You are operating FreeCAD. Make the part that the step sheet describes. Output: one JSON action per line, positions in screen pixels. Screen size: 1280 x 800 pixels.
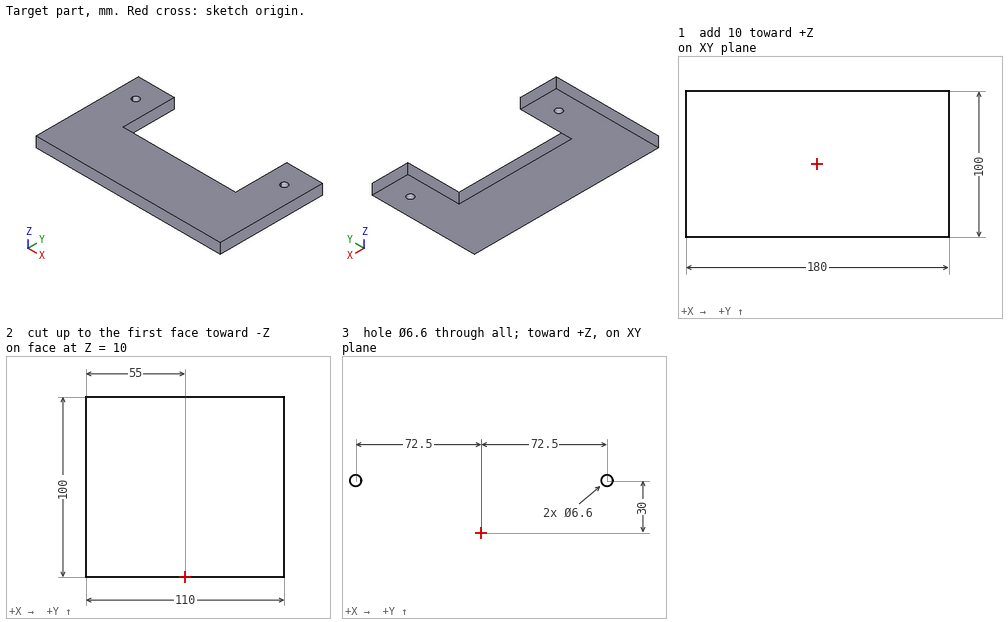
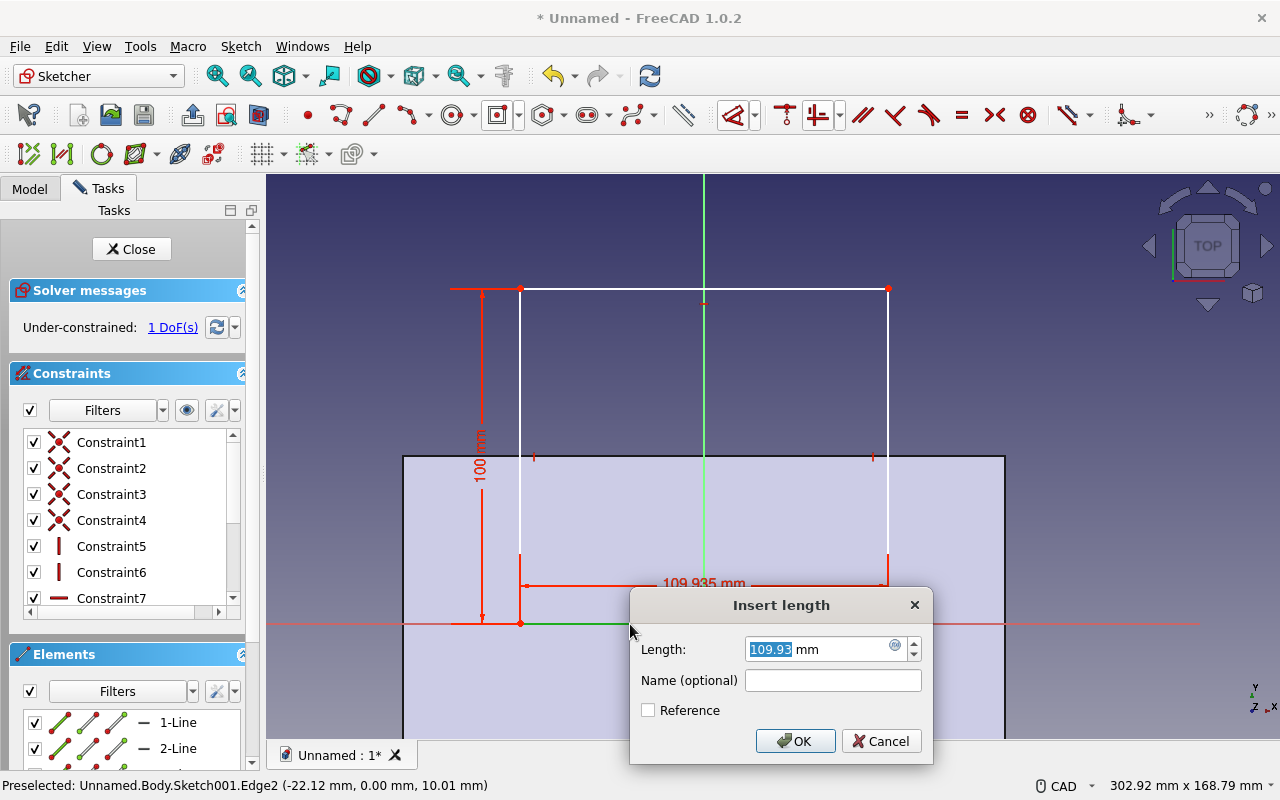
{"action": "type", "text": "110"}
{"action": "key", "text": "Return"}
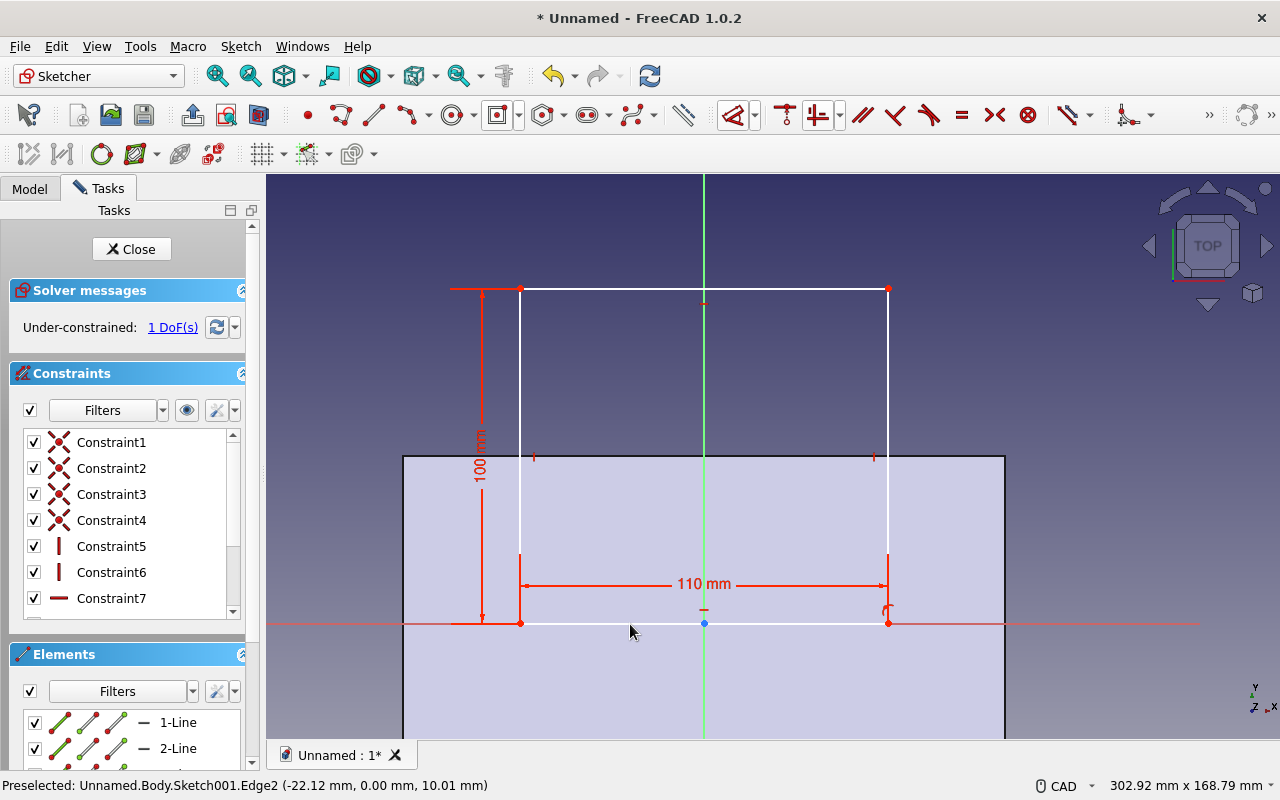
{"action": "left_click", "coordinate": [520, 289]}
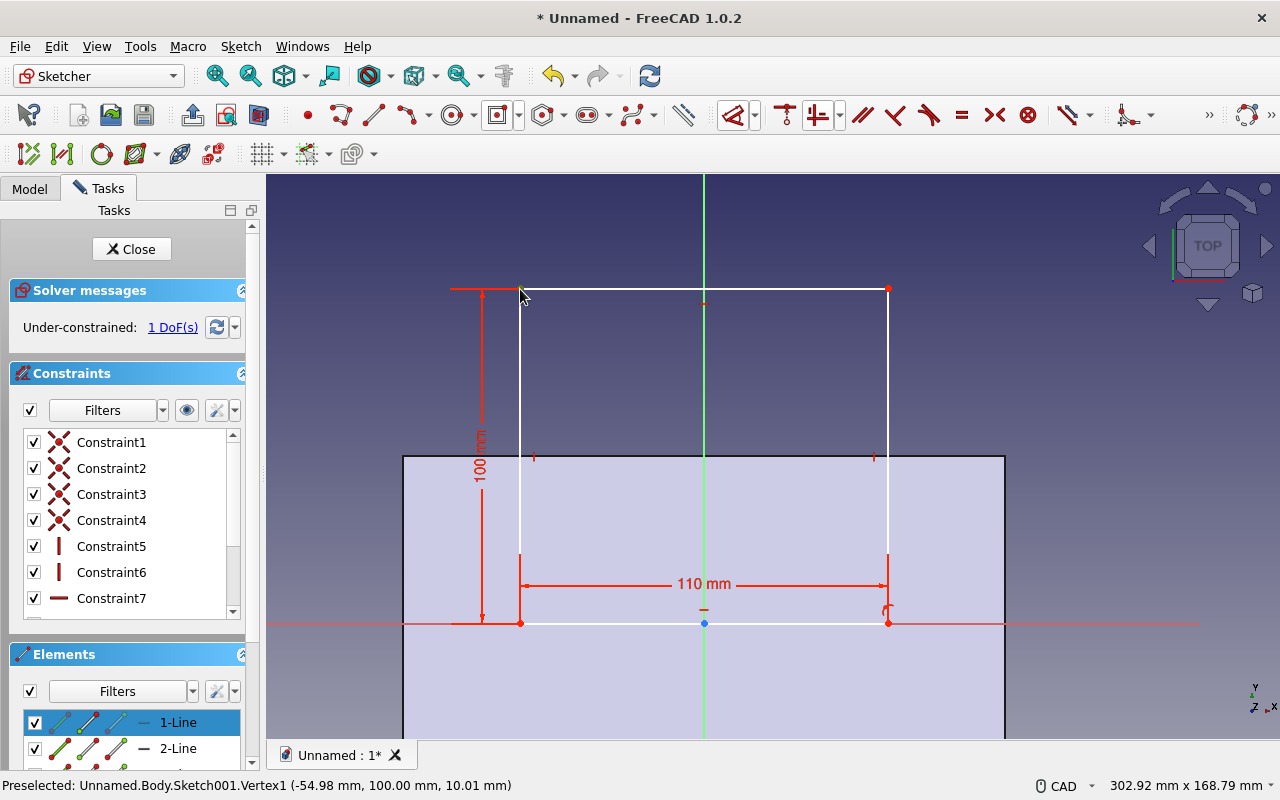
{"action": "key", "text": "l"}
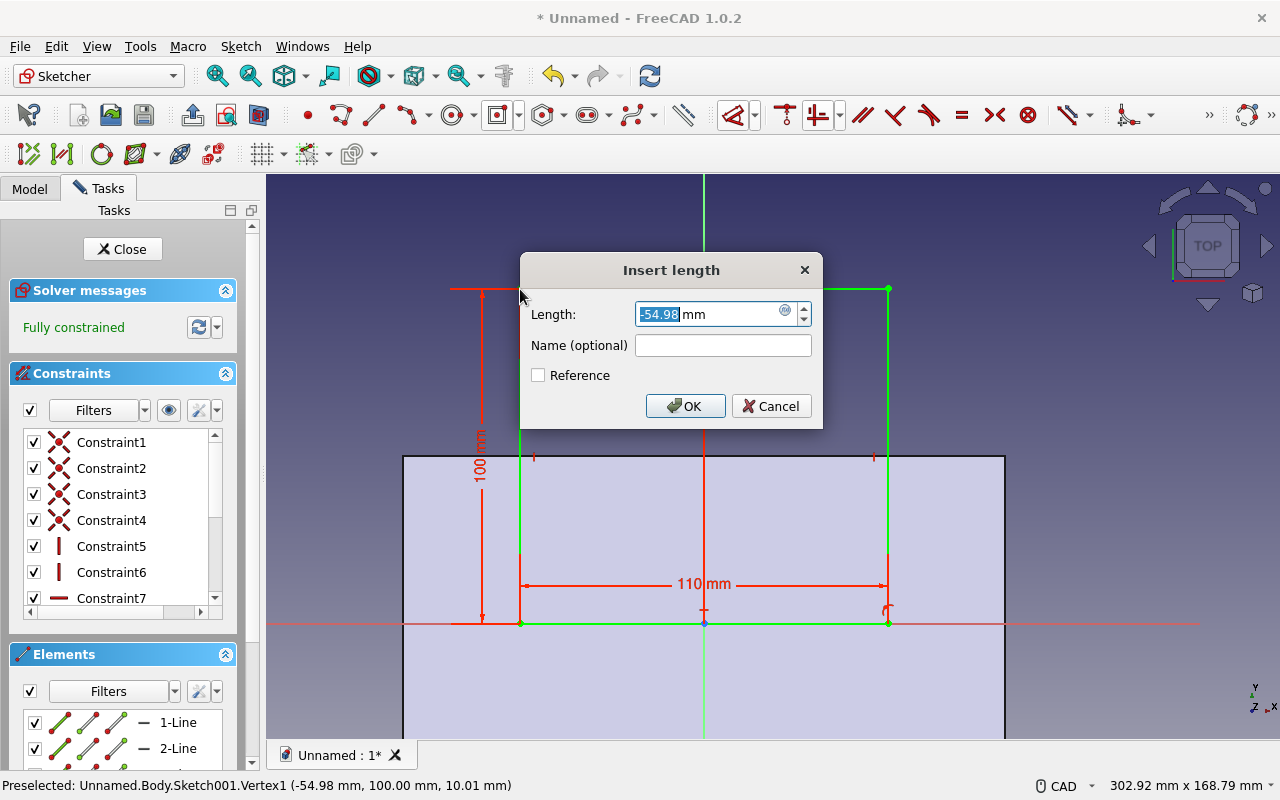
{"action": "type", "text": "-55"}
{"action": "key", "text": "Return"}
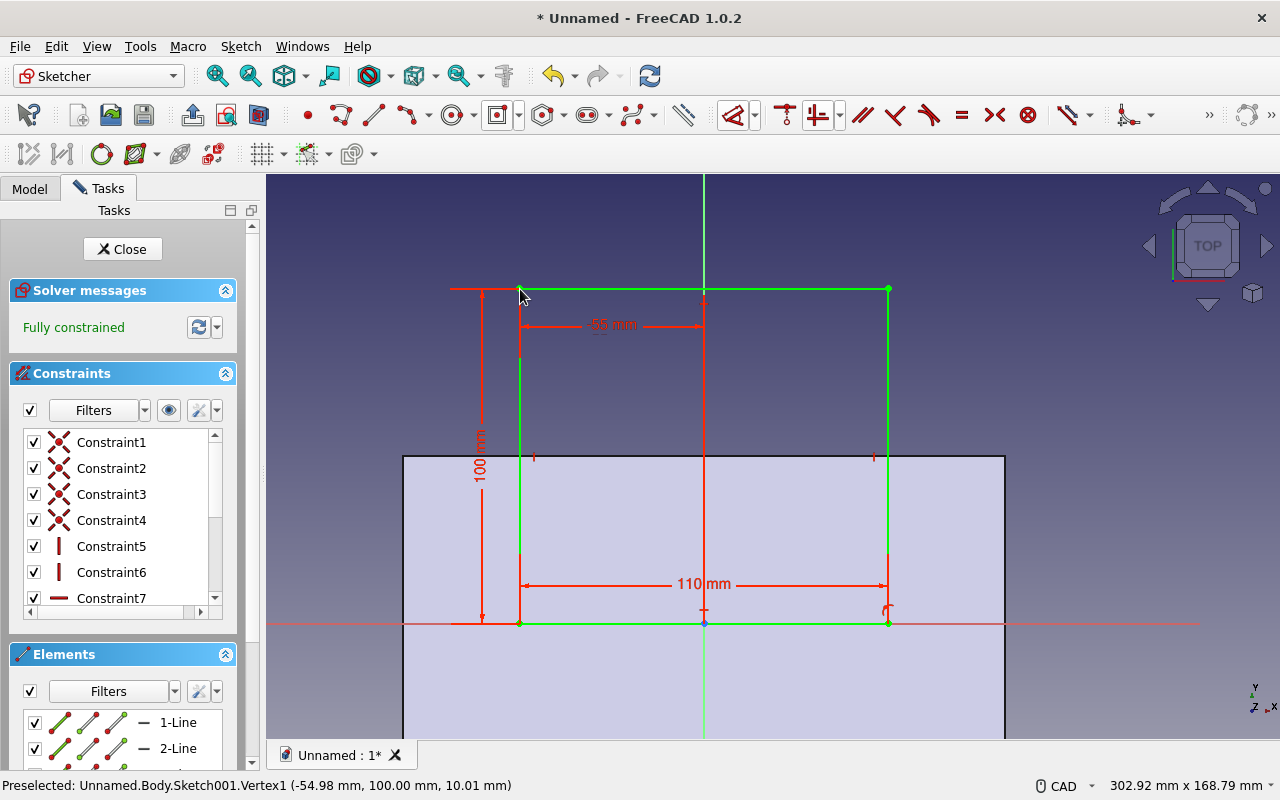
{"action": "left_click", "coordinate": [123, 249]}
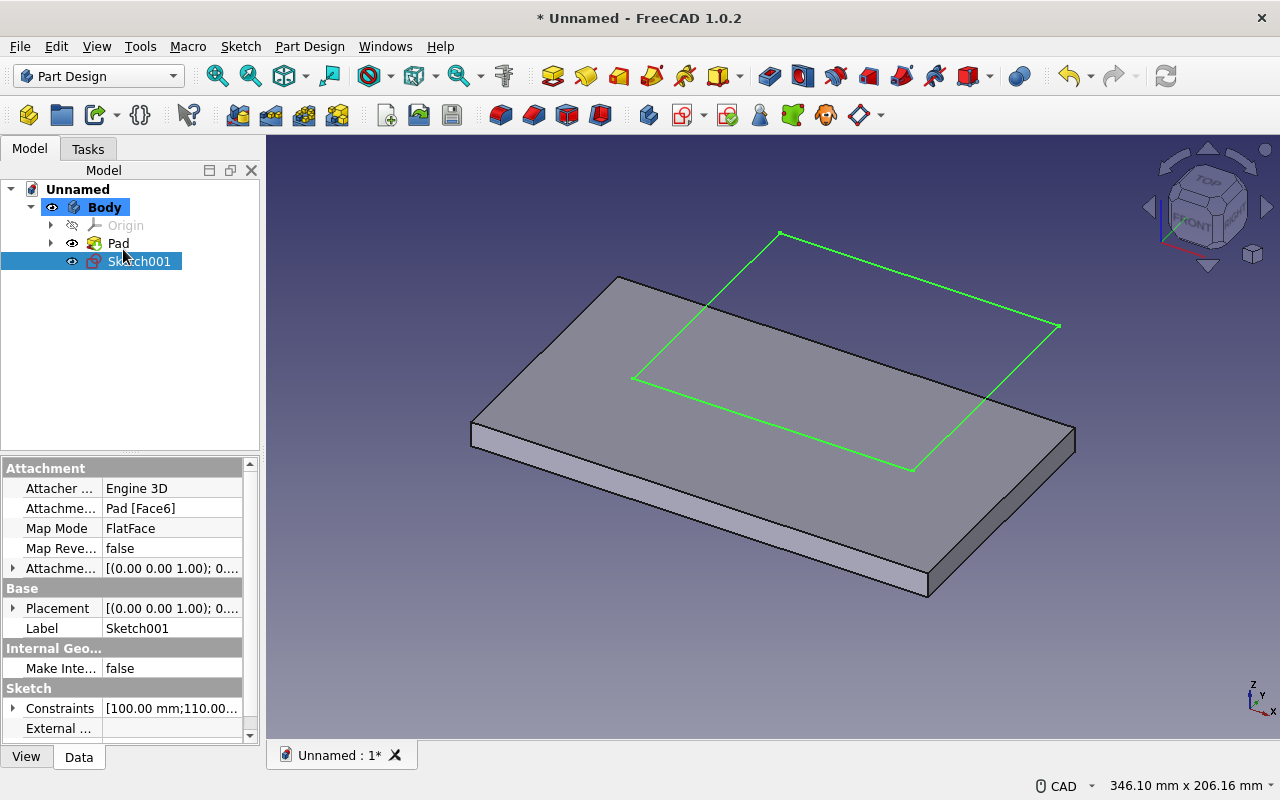
{"action": "left_click", "coordinate": [770, 76]}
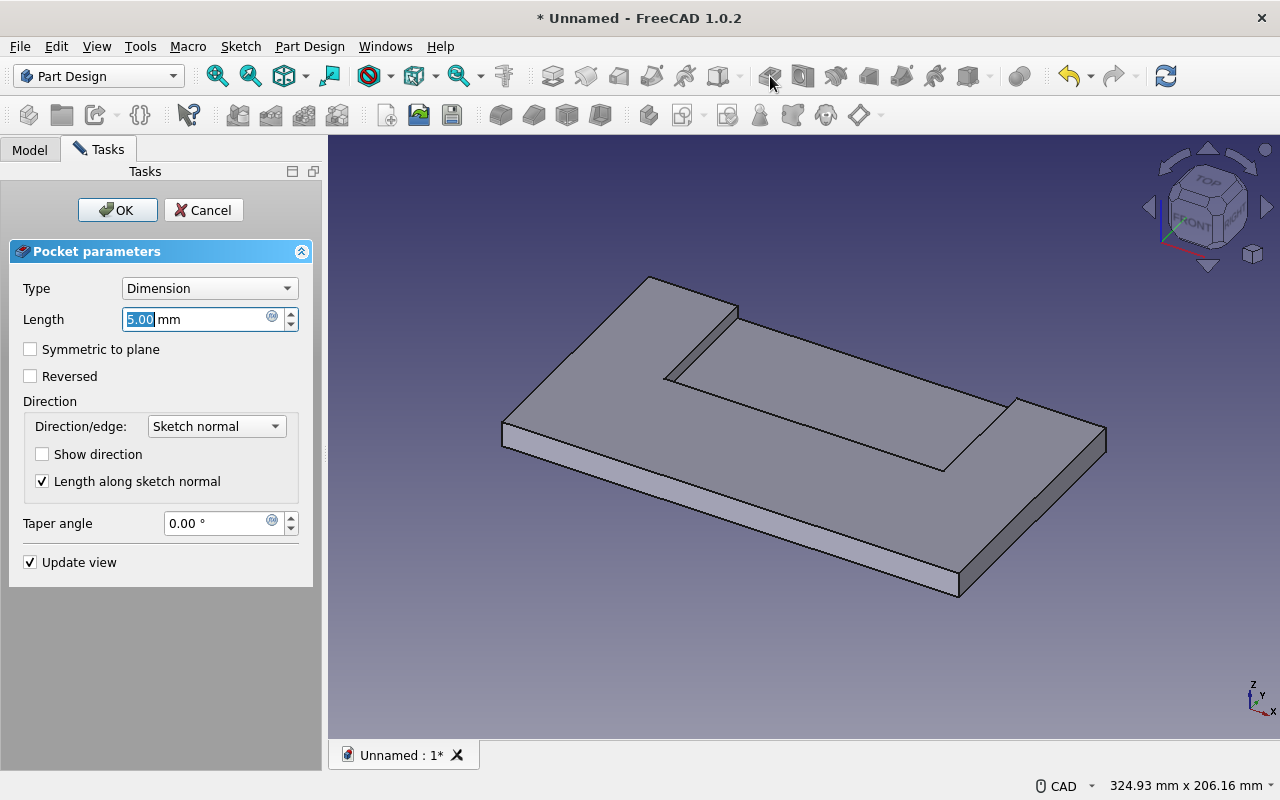
{"action": "left_click", "coordinate": [210, 288]}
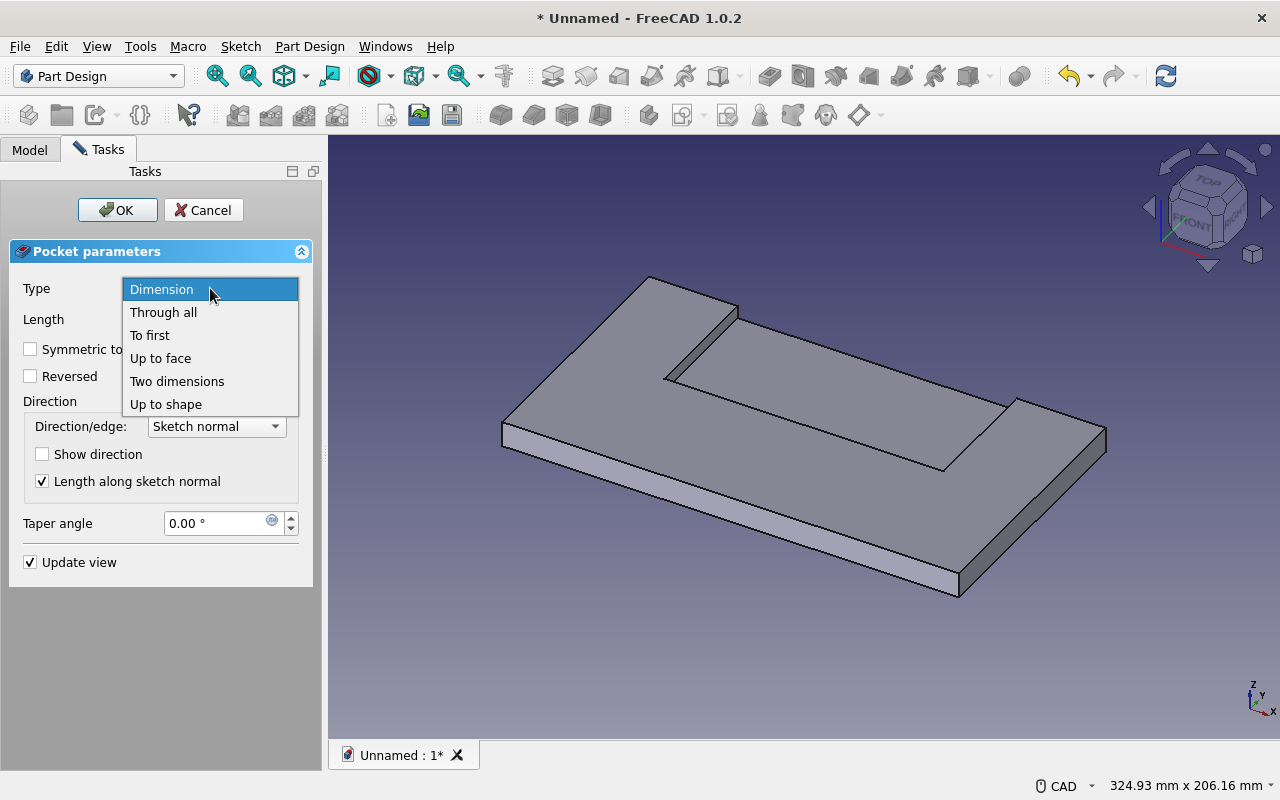
{"action": "left_click", "coordinate": [208, 336]}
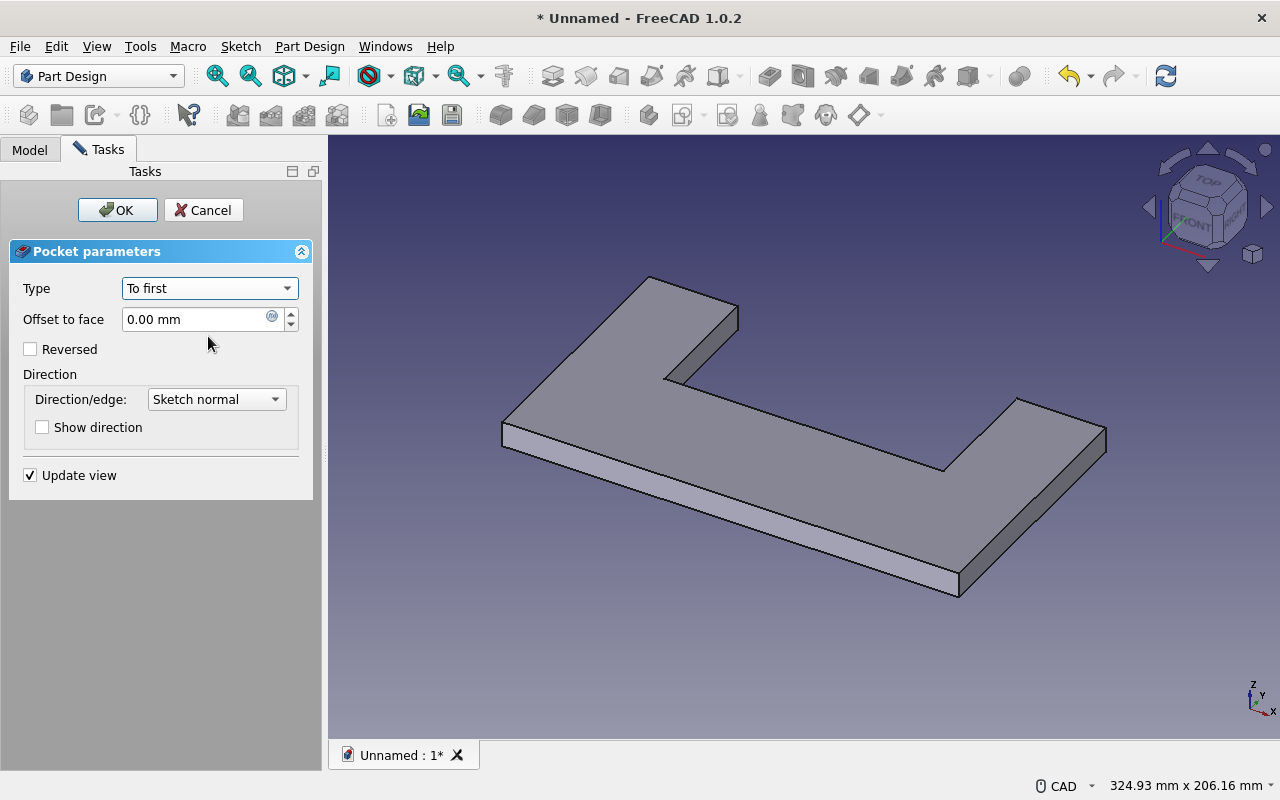
{"action": "left_click", "coordinate": [118, 210]}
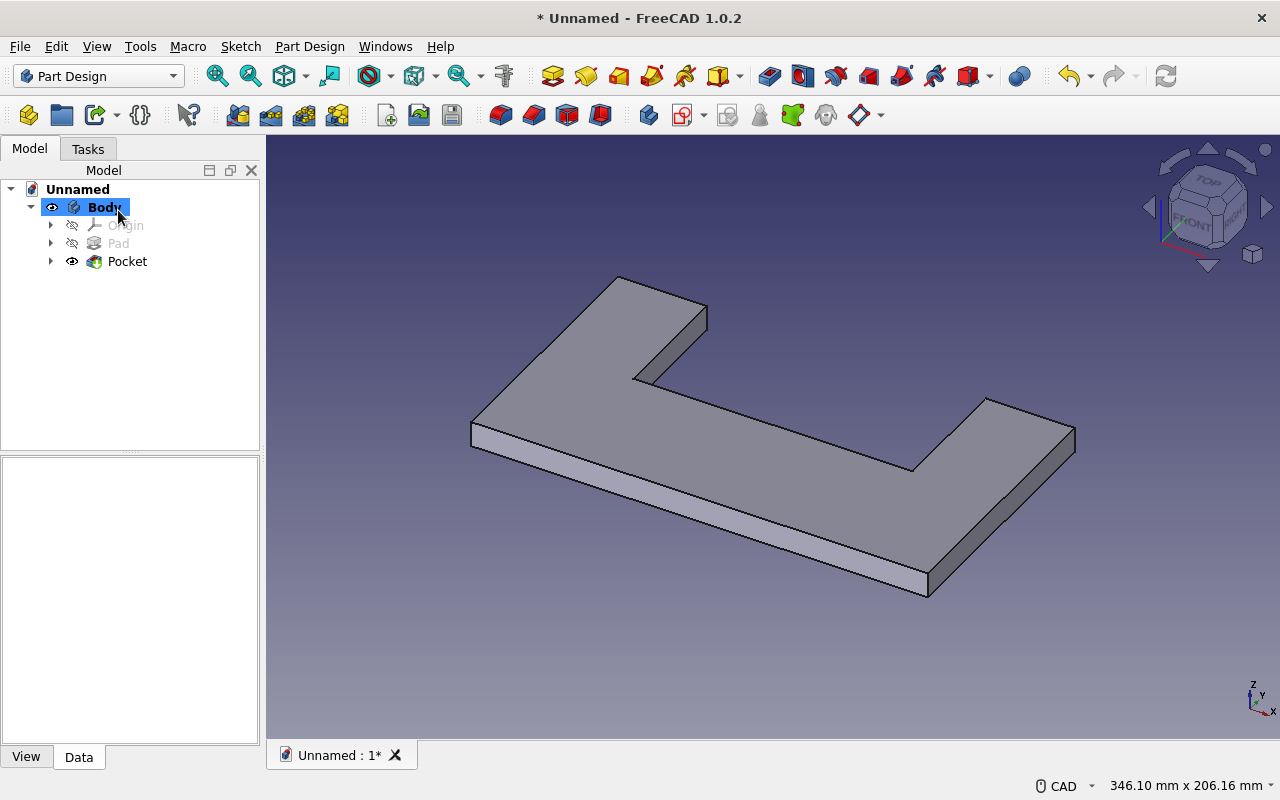
{"action": "left_click", "coordinate": [682, 116]}